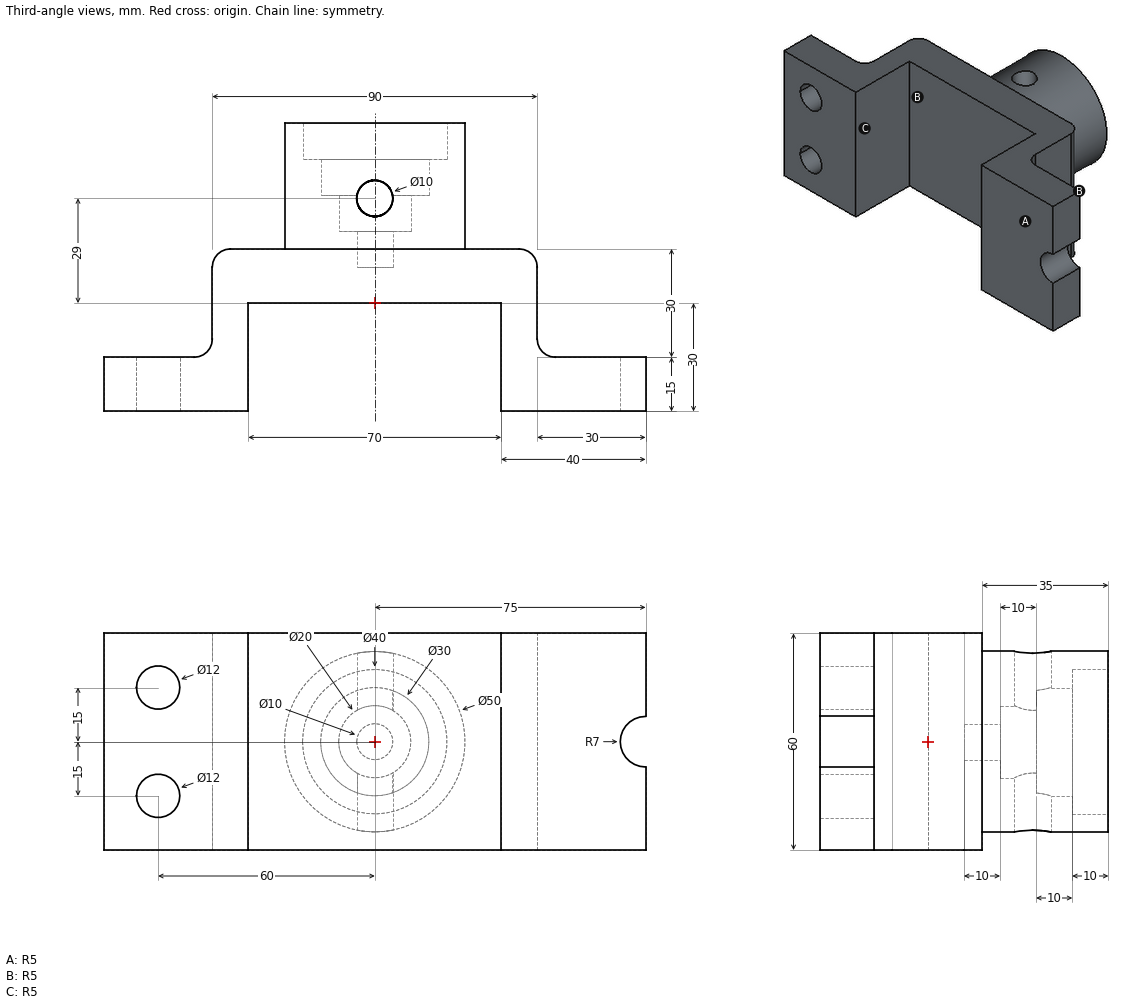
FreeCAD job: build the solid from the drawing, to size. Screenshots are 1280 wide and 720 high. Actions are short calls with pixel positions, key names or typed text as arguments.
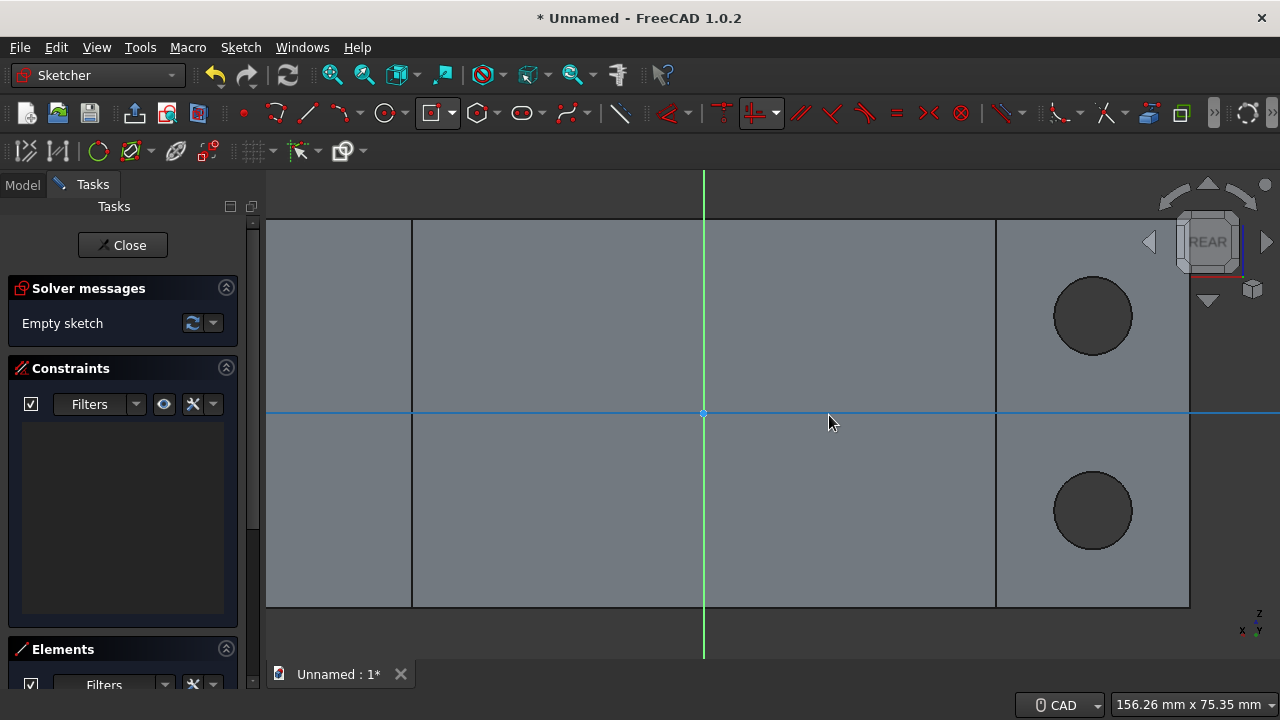
click(386, 114)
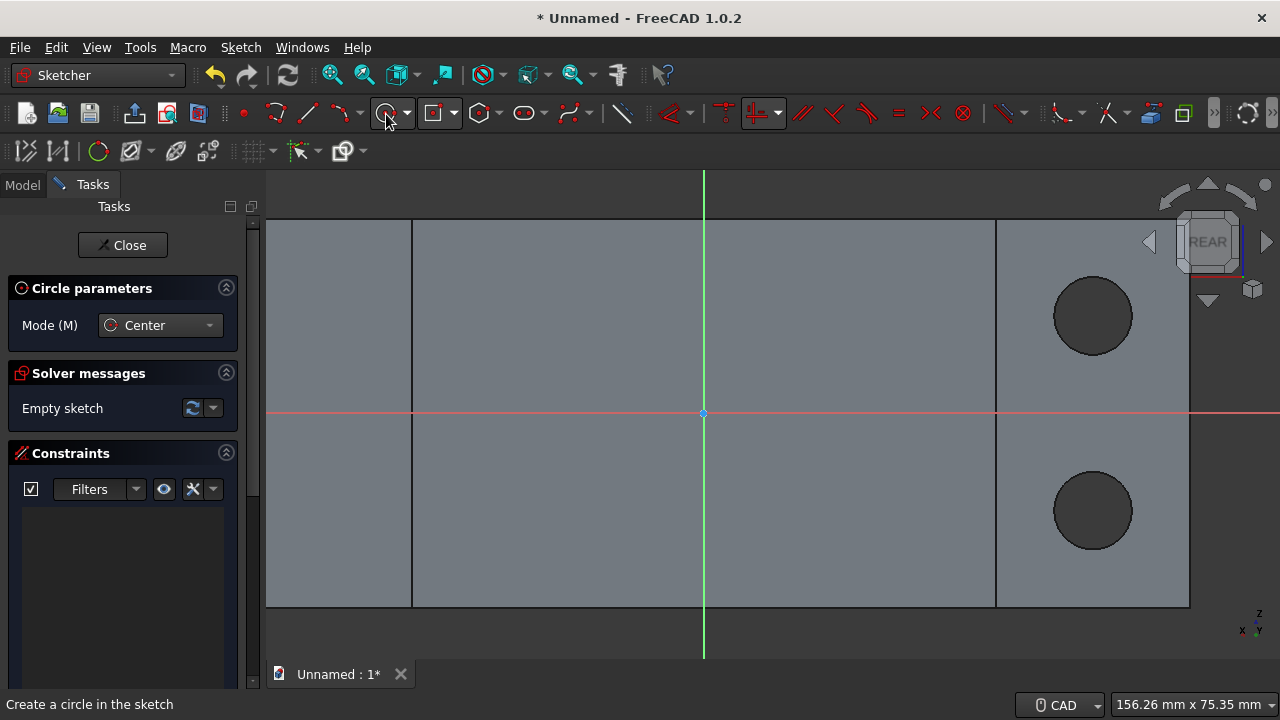
click(704, 413)
click(818, 299)
key(Escape)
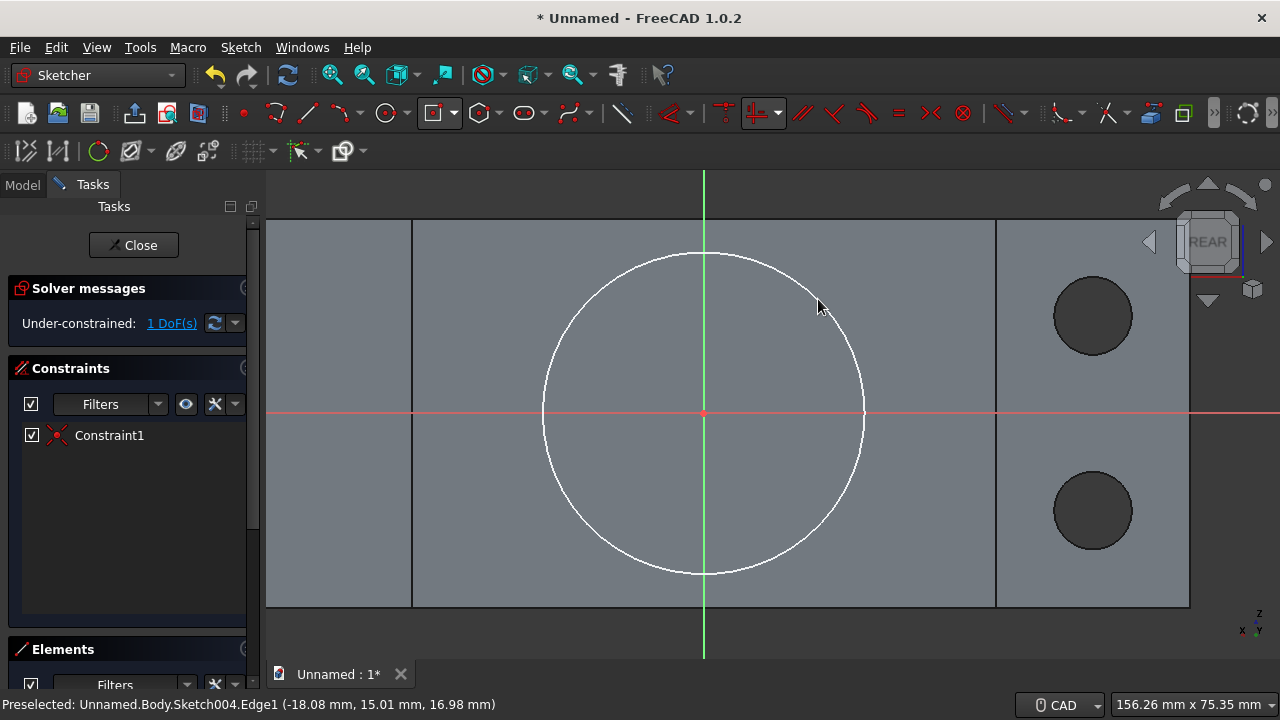
click(670, 114)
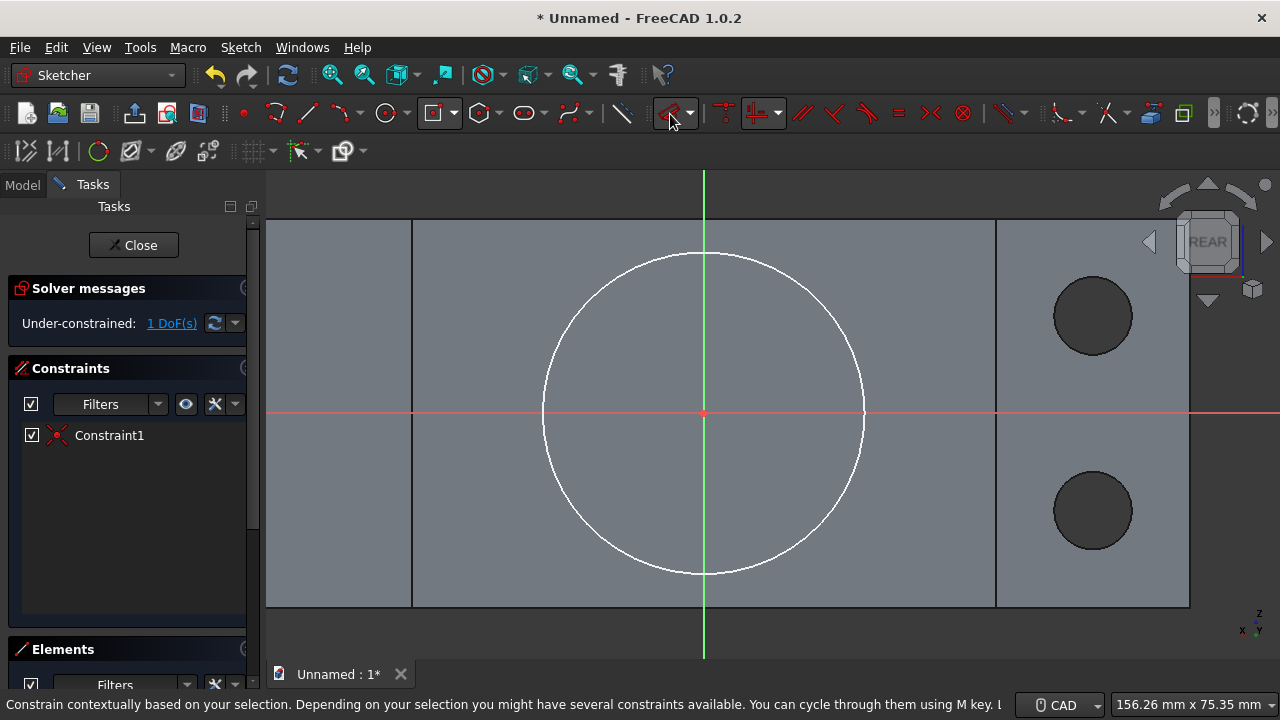
click(817, 299)
click(840, 276)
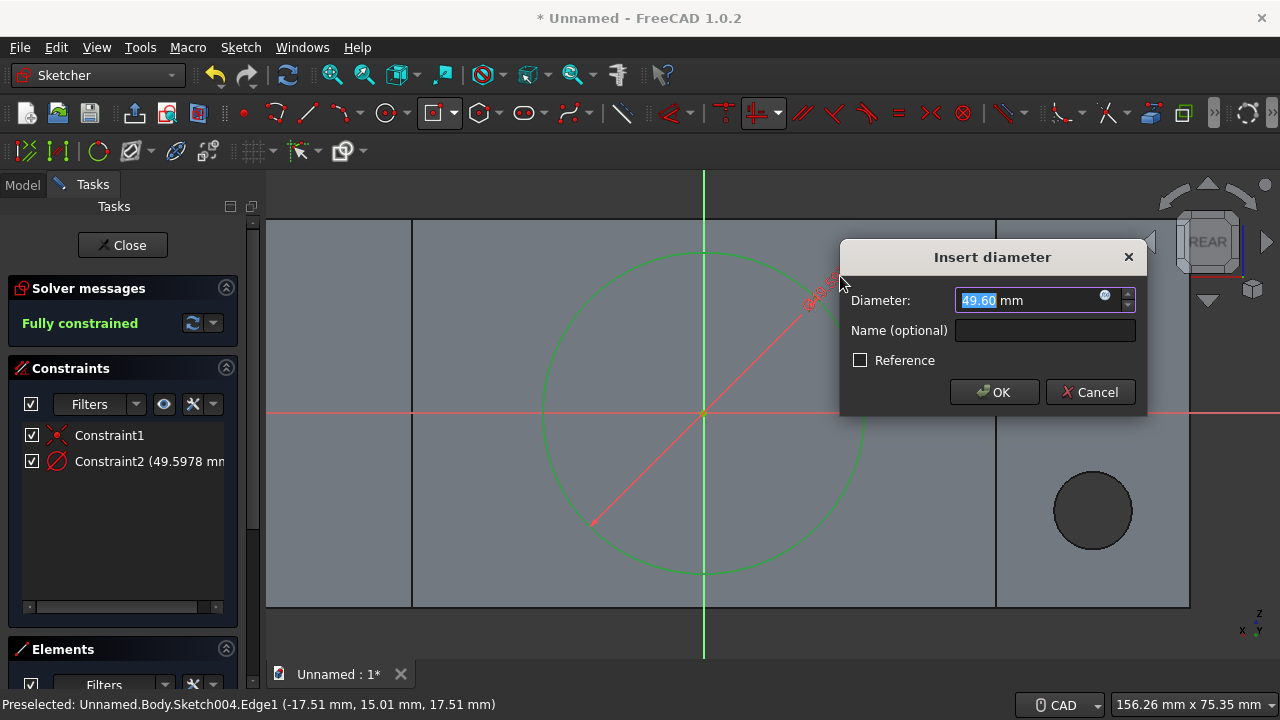
text(50)
key(Return)
key(Escape)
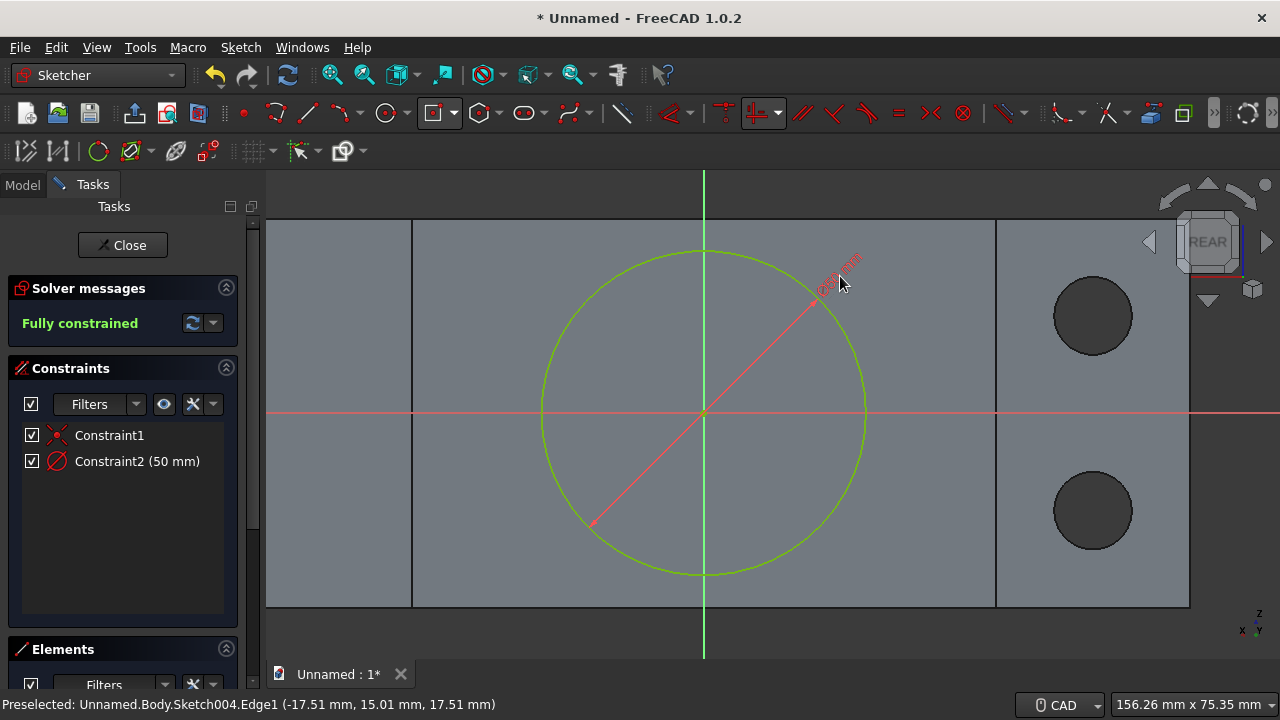
click(123, 245)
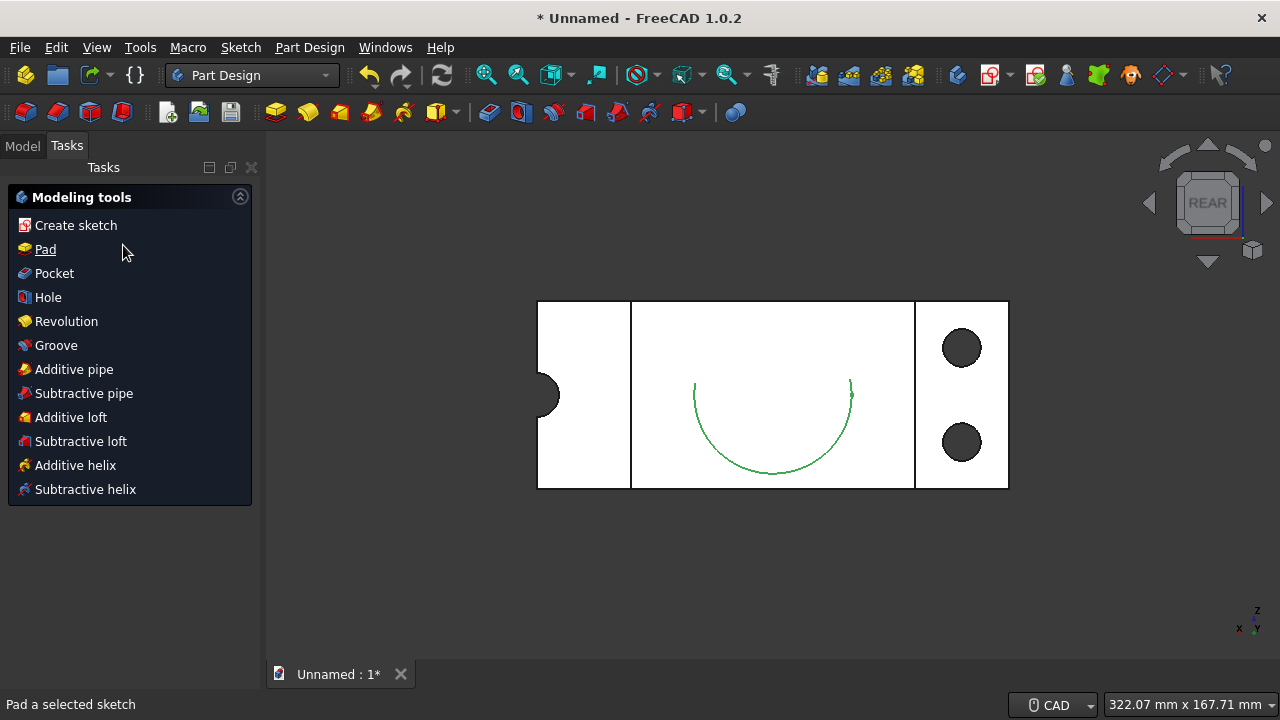
click(276, 112)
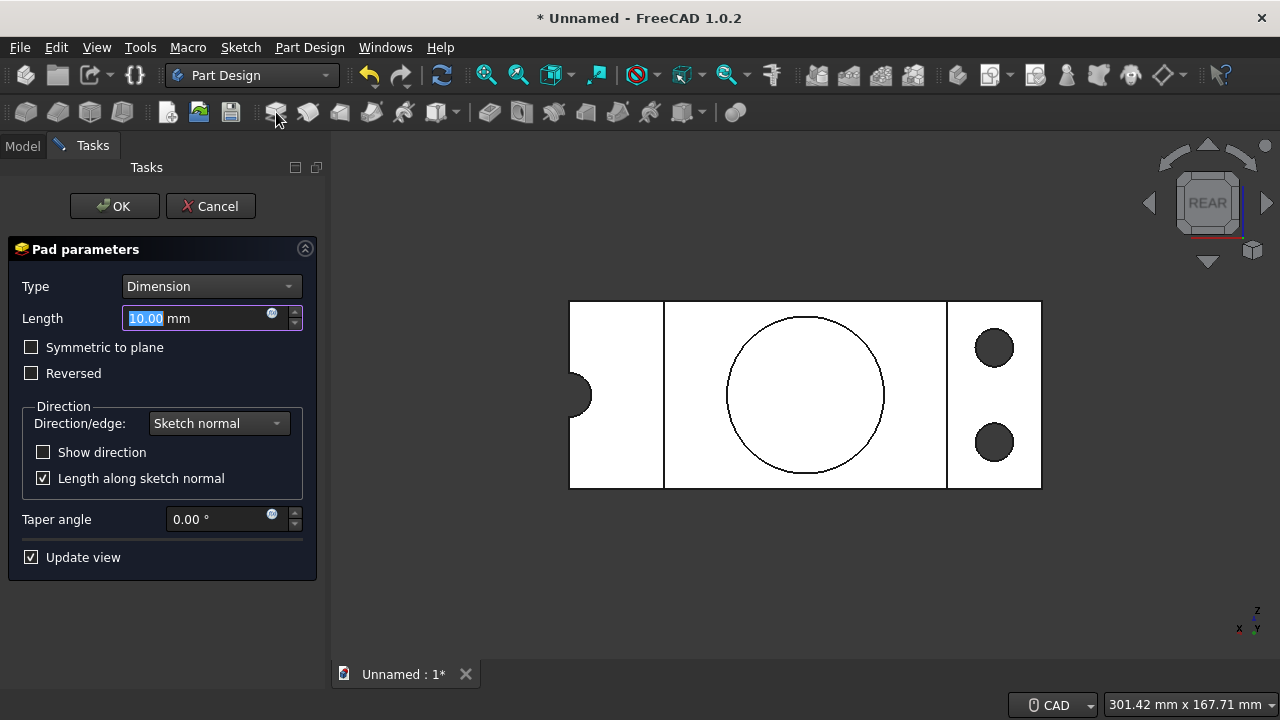
text(35)
key(Tab)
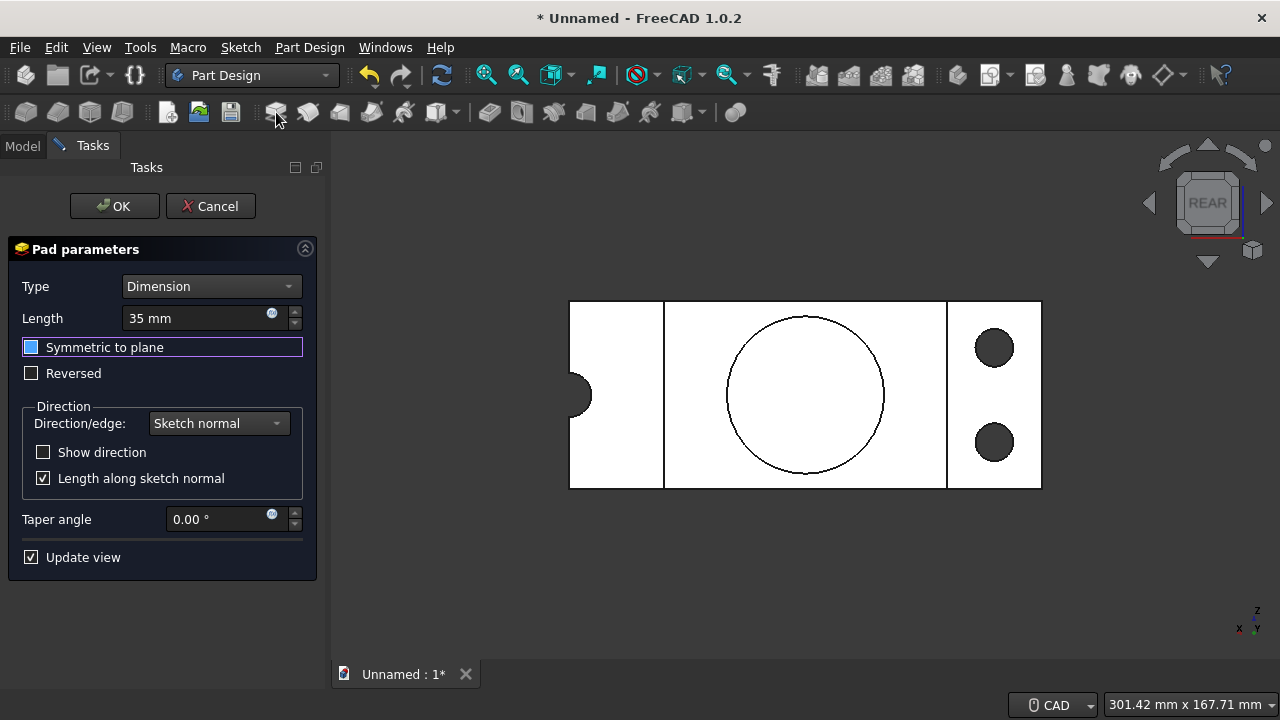
click(115, 206)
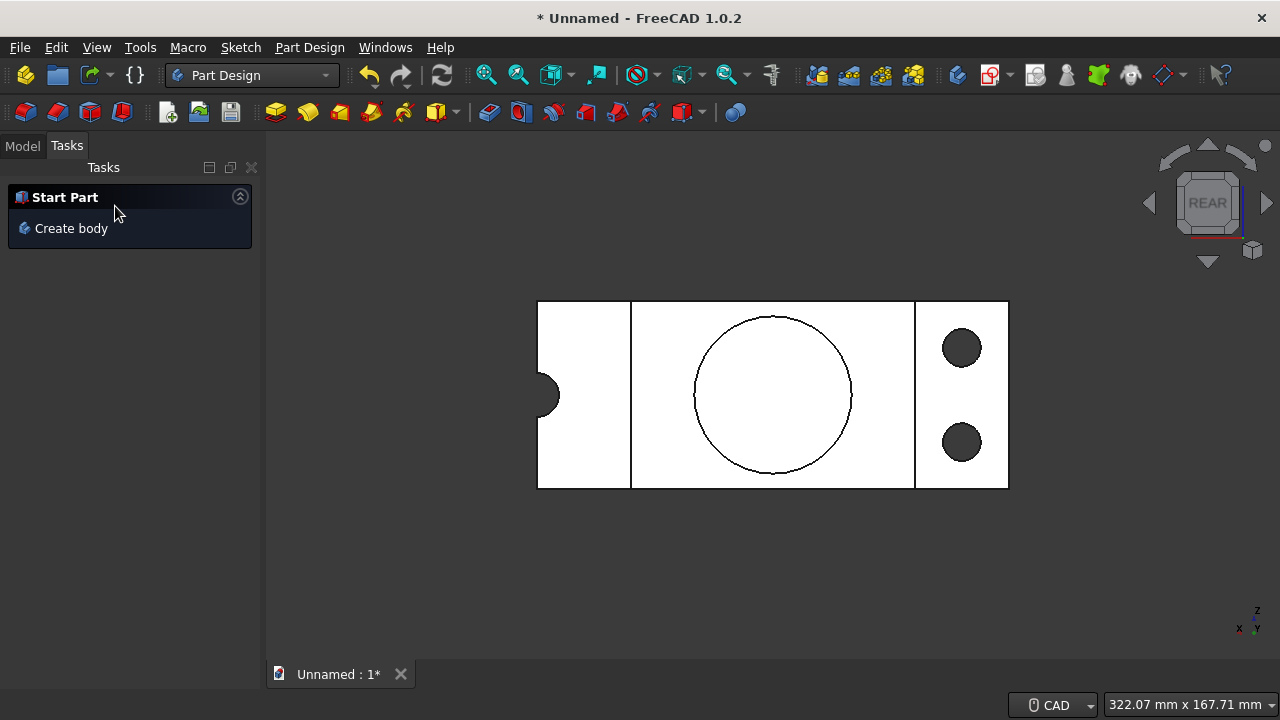
click(773, 394)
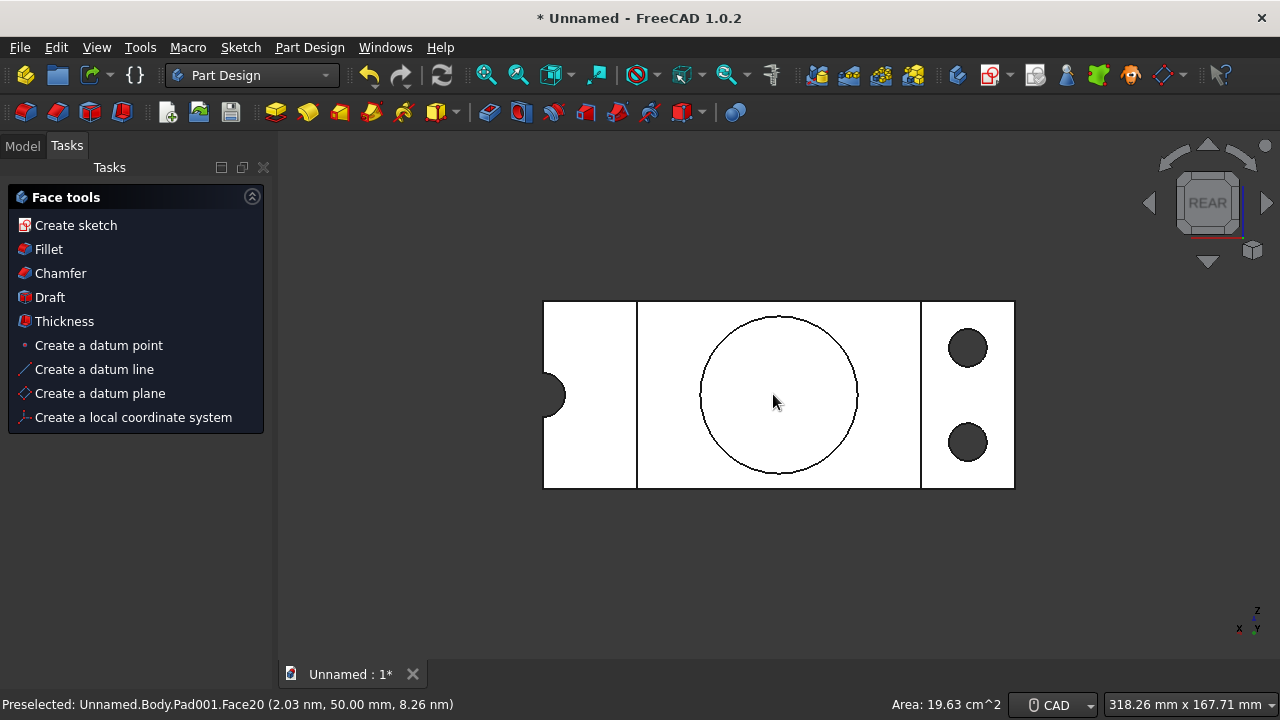
click(990, 76)